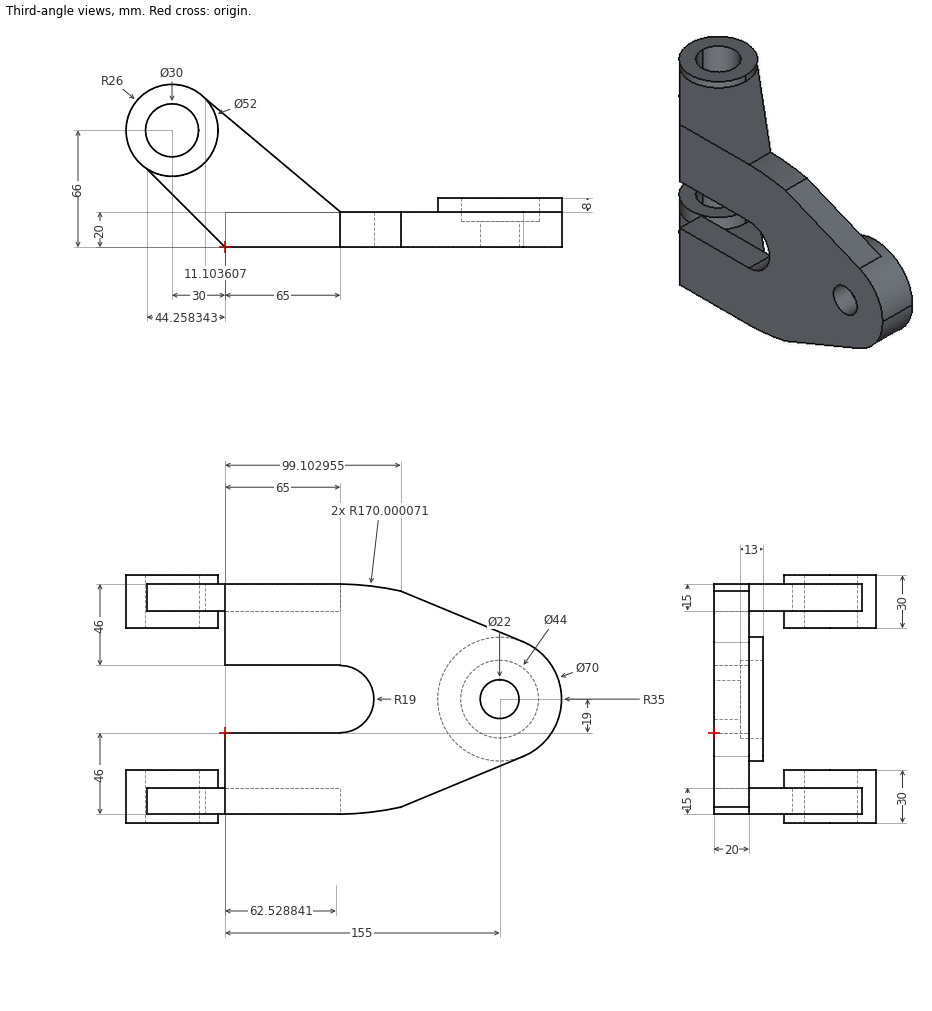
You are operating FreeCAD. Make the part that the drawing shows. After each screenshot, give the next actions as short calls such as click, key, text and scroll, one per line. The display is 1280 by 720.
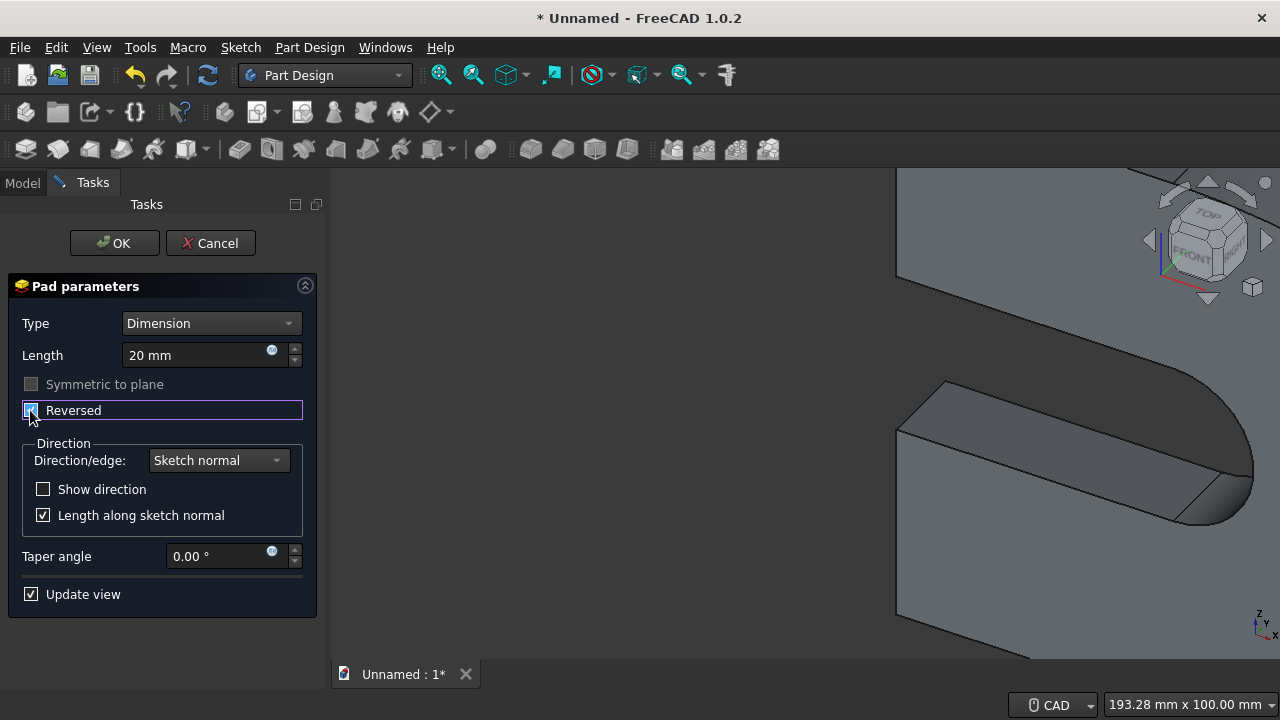
click(115, 243)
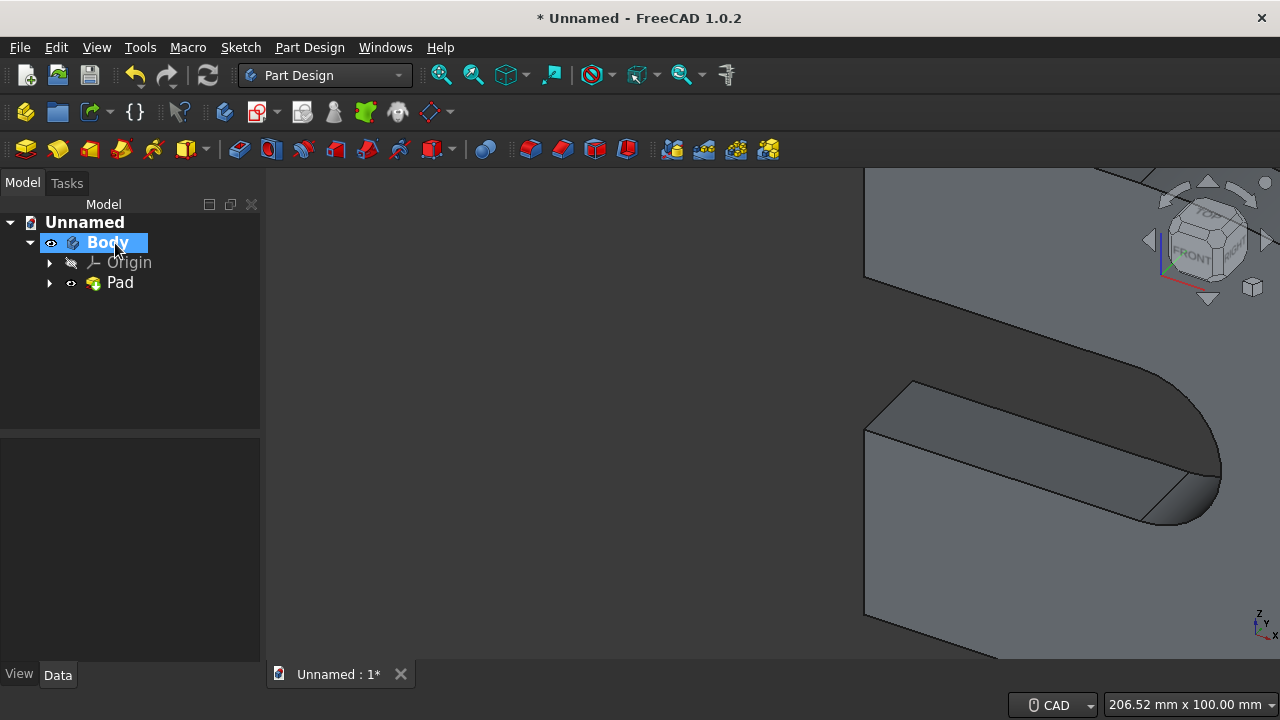
key(v)
key(f)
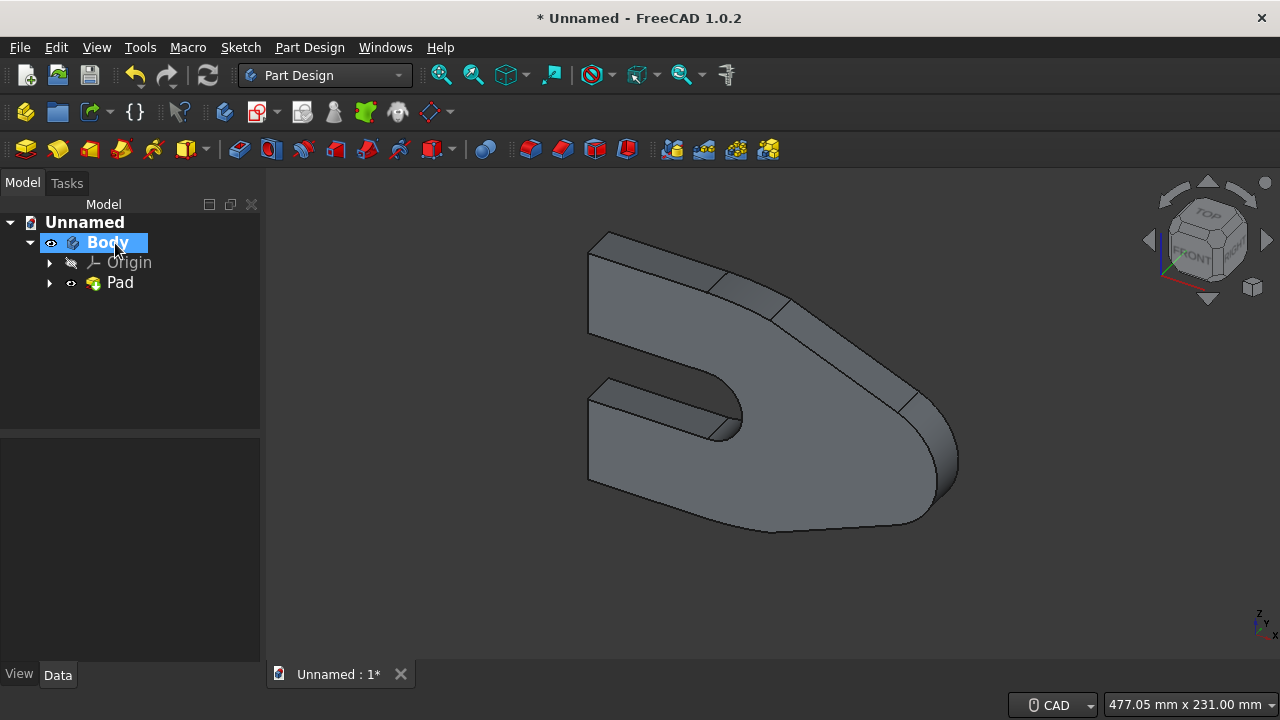
key(4)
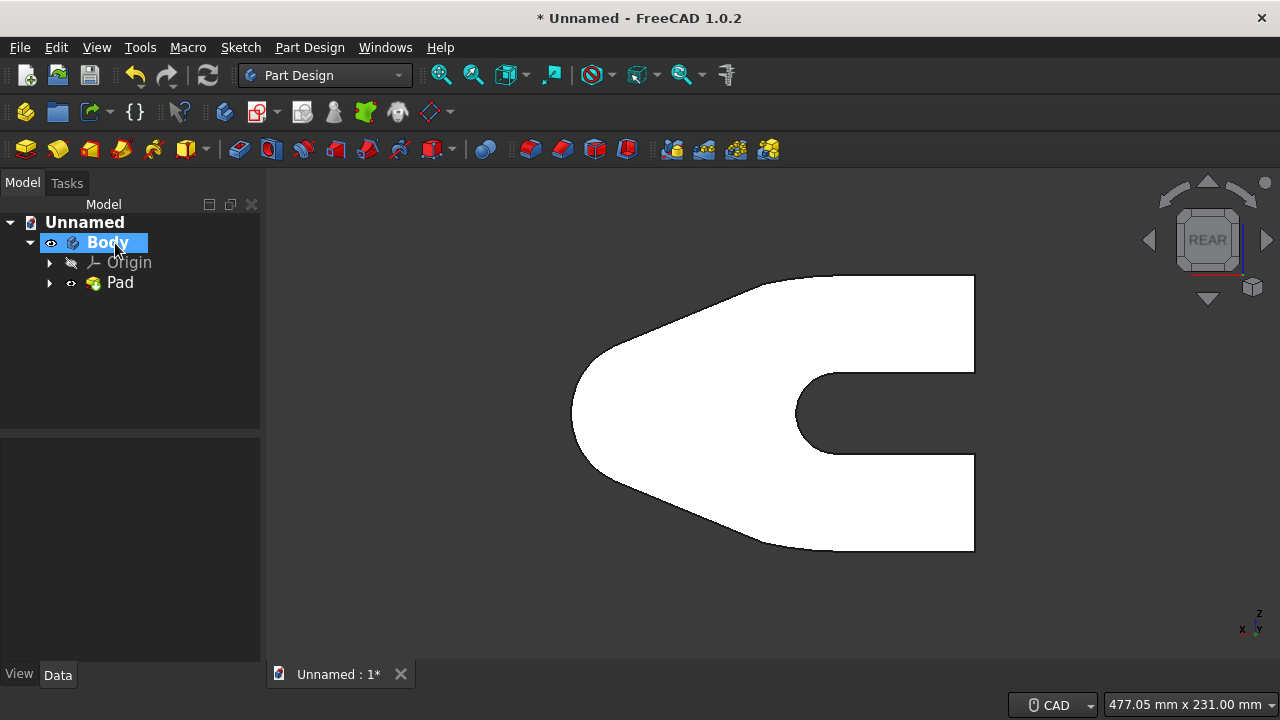
click(715, 412)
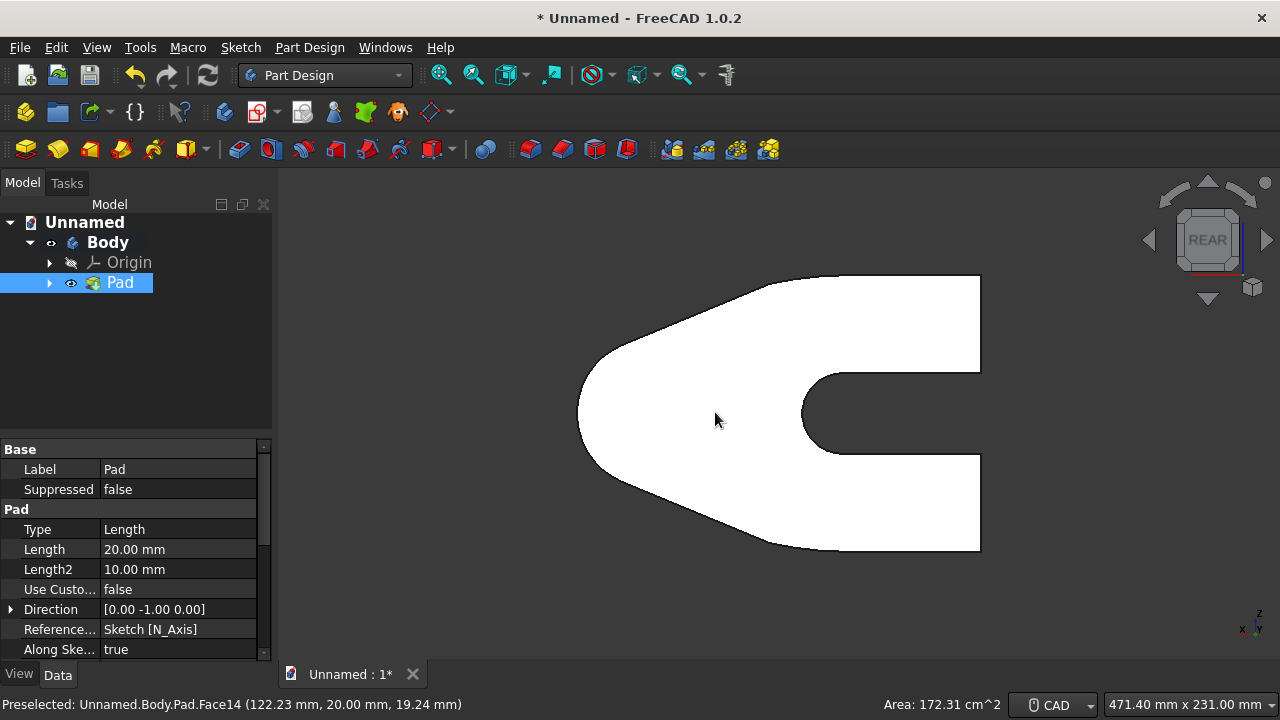
click(258, 112)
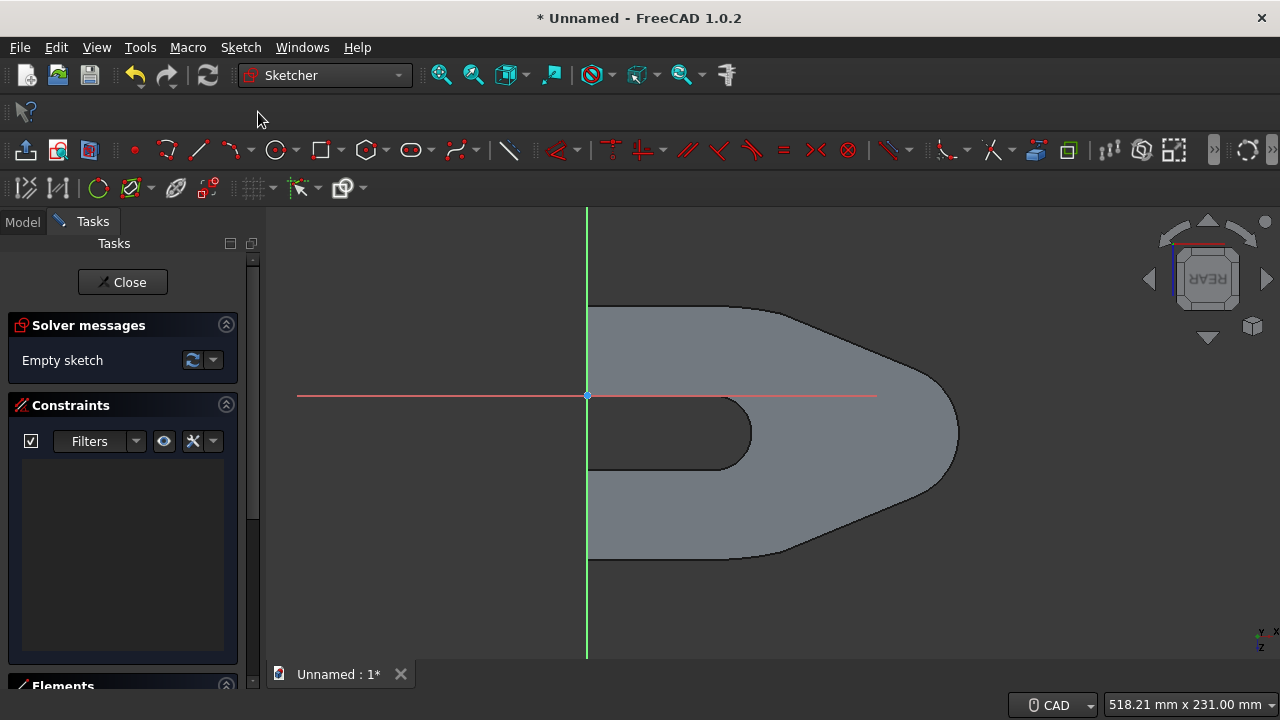
scroll(1042, 433, up, 4)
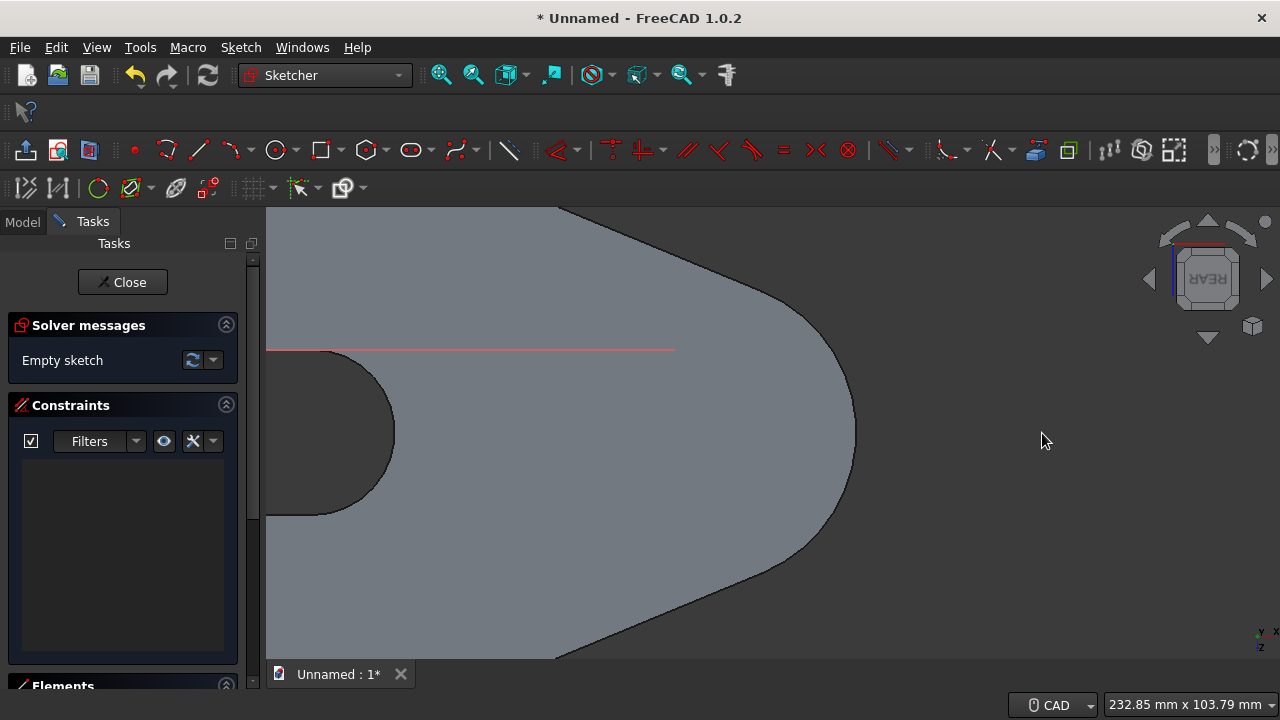
key(g)
key(c)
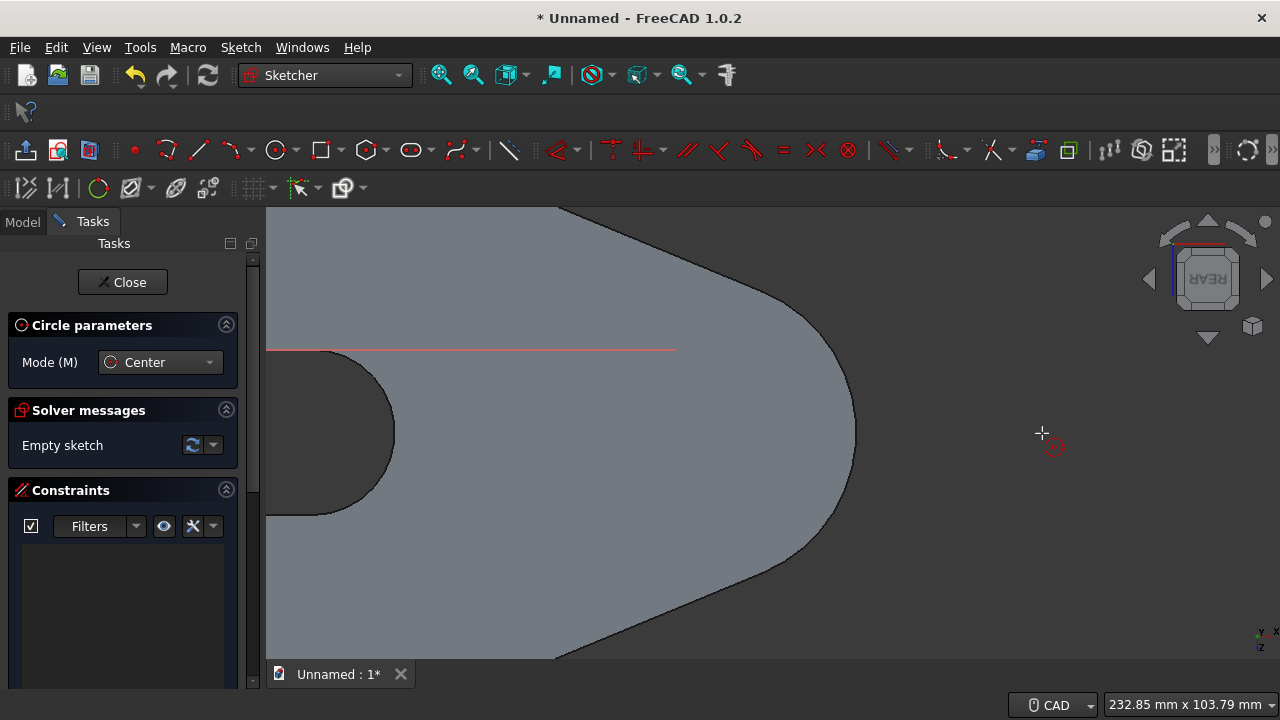
click(704, 432)
move(812, 325)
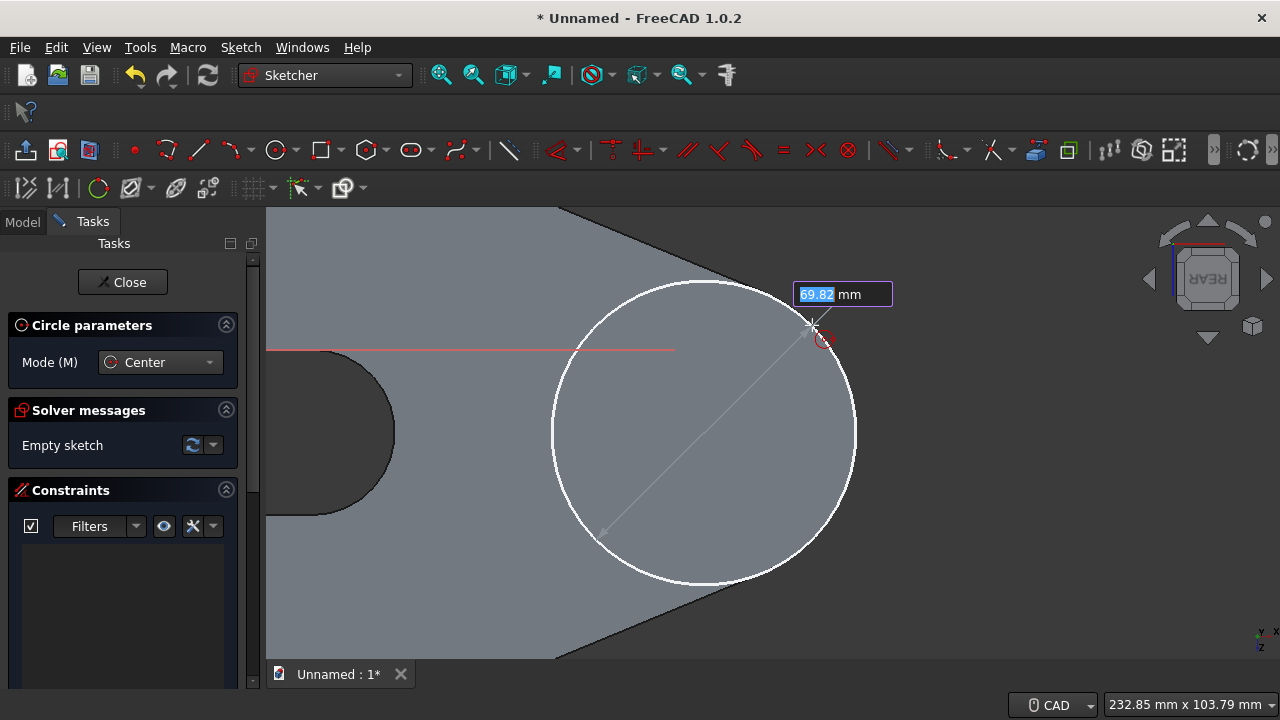
text(70)
key(Return)
key(Escape)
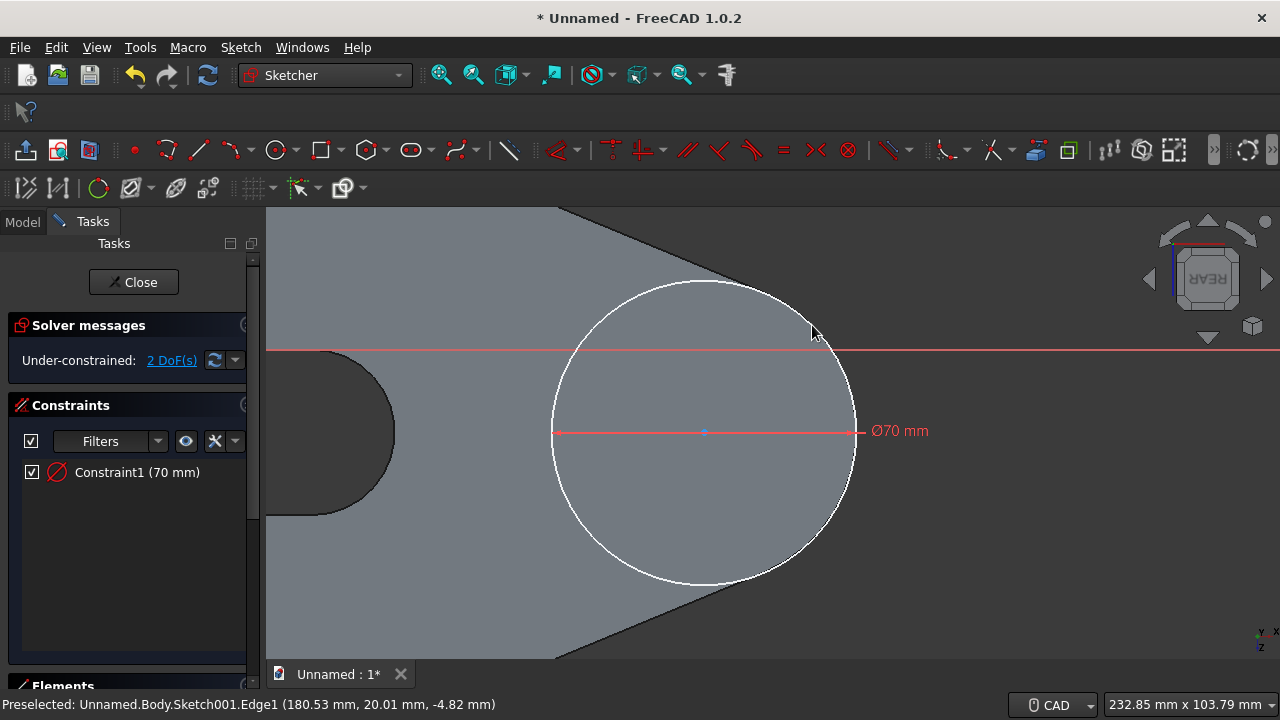
key(d)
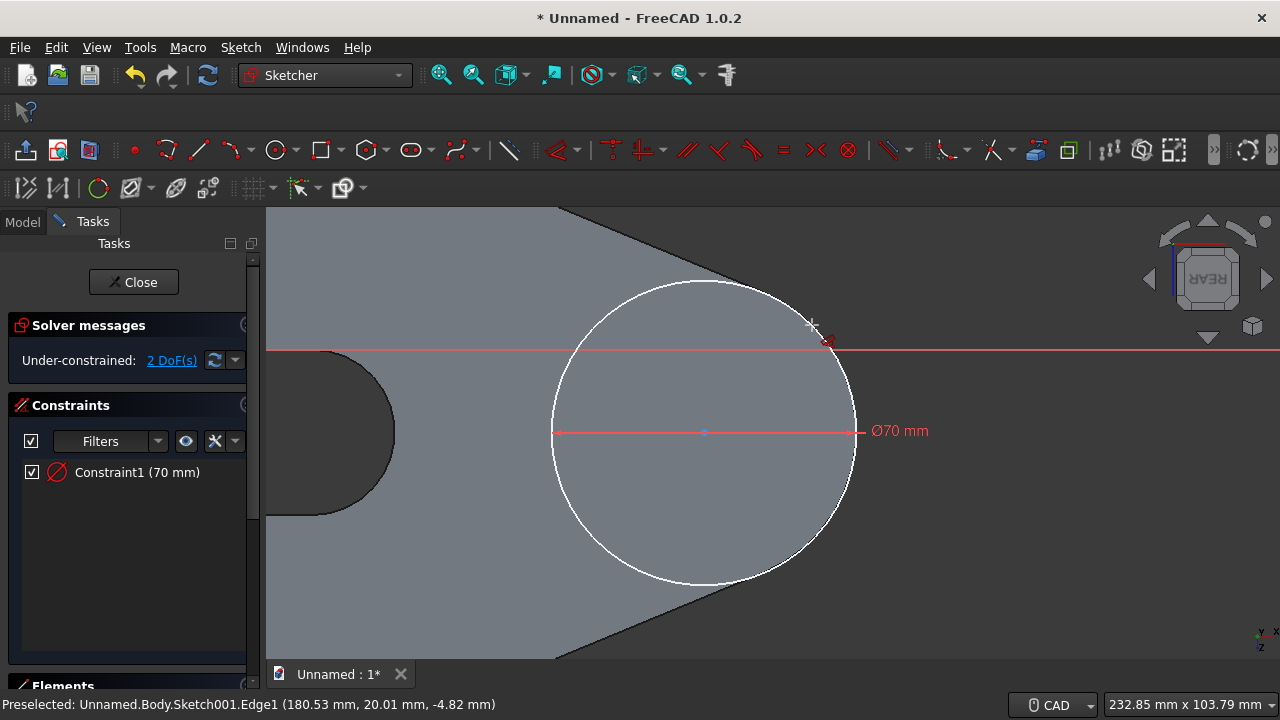
click(704, 433)
click(738, 391)